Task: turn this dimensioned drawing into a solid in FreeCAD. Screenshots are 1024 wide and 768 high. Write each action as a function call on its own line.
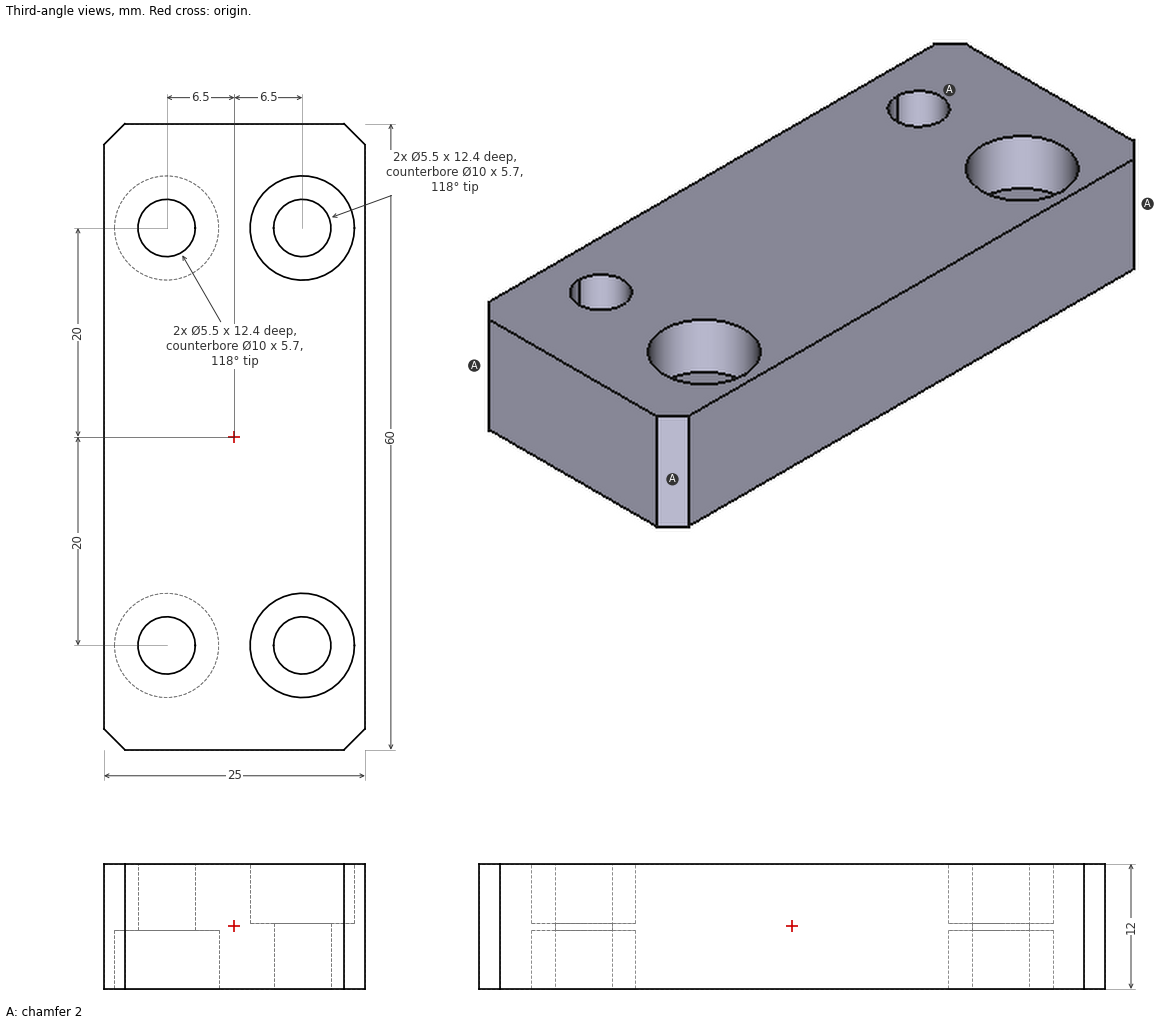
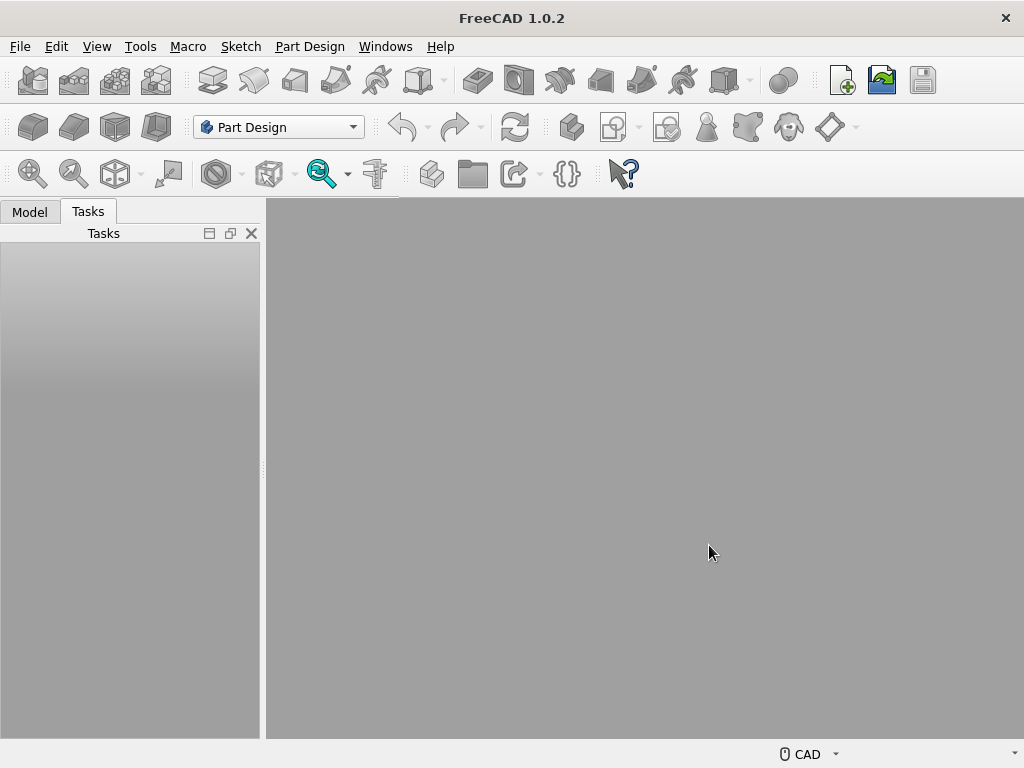
click(841, 80)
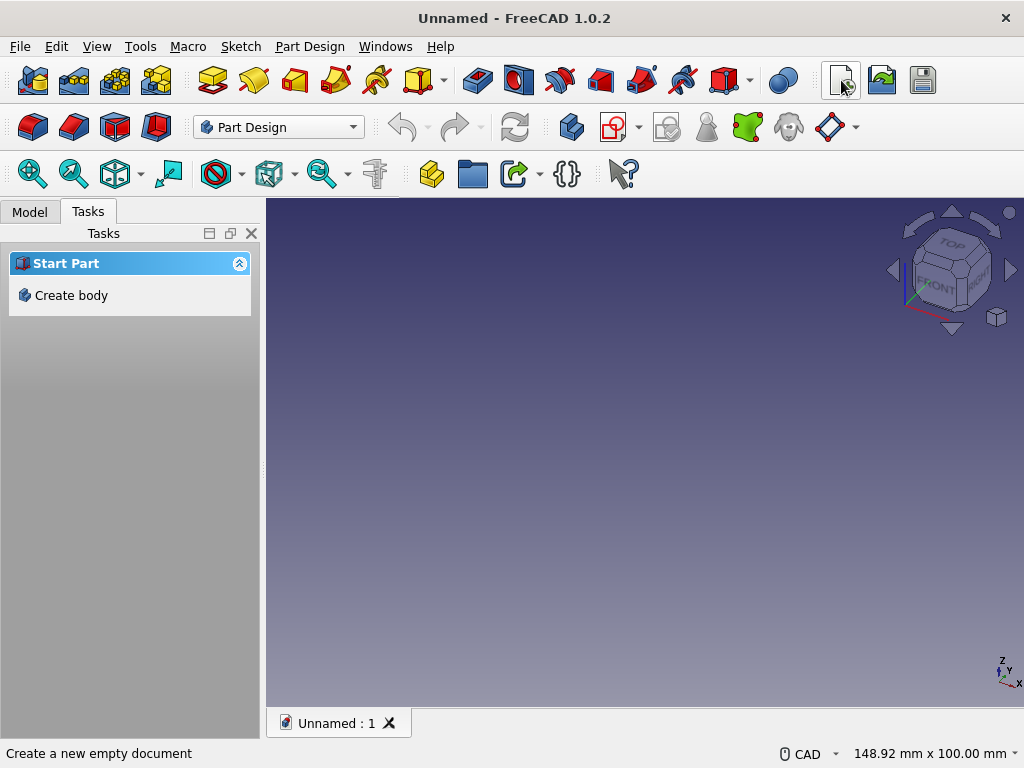
click(612, 128)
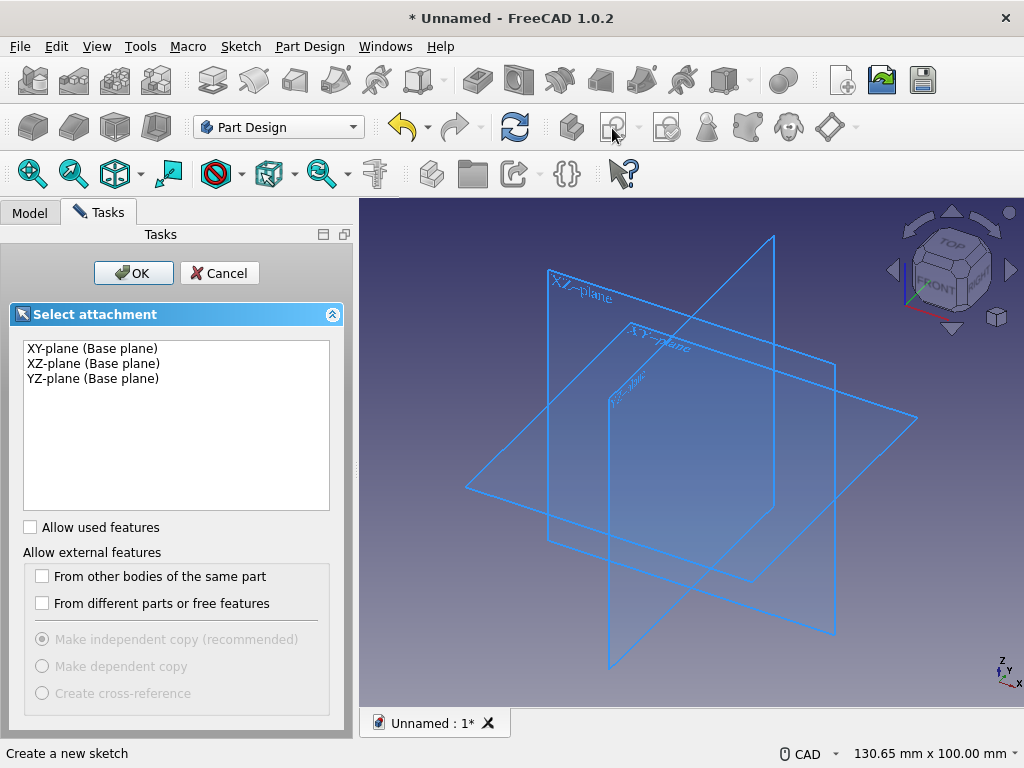
click(84, 348)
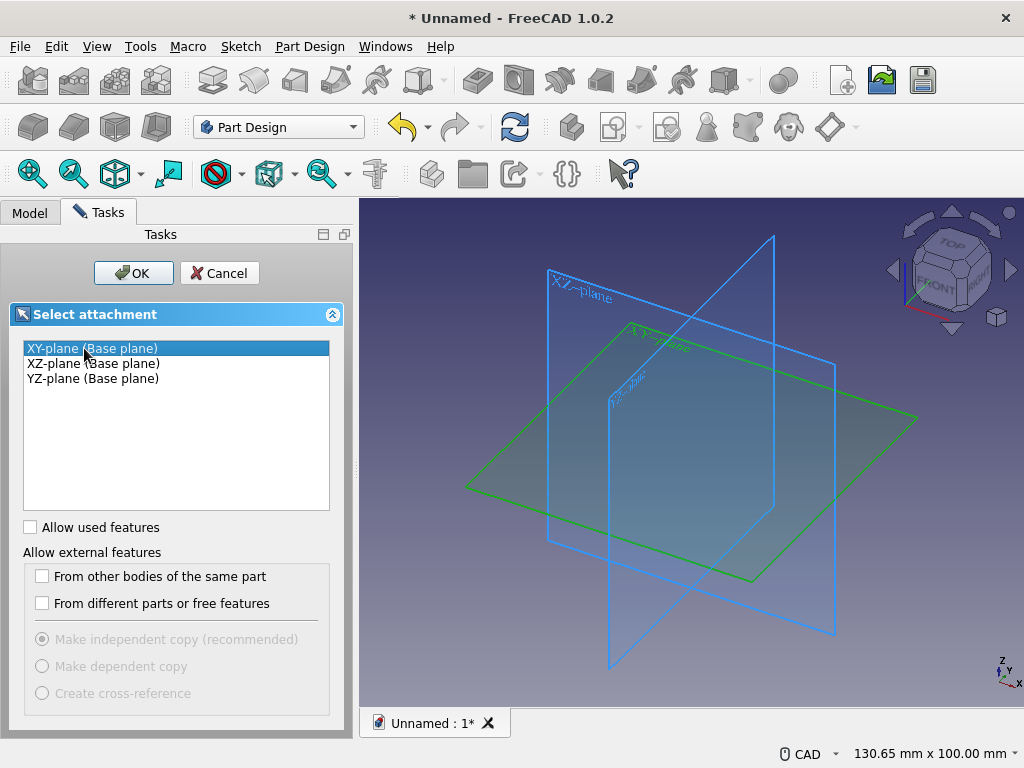
click(134, 273)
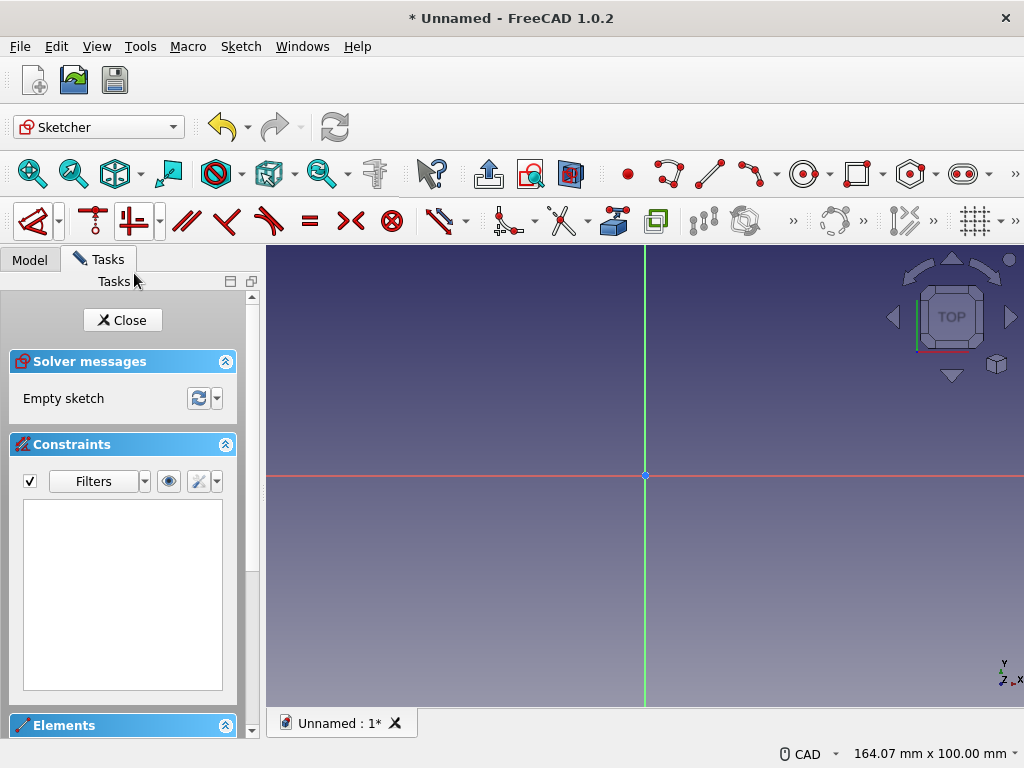
click(882, 174)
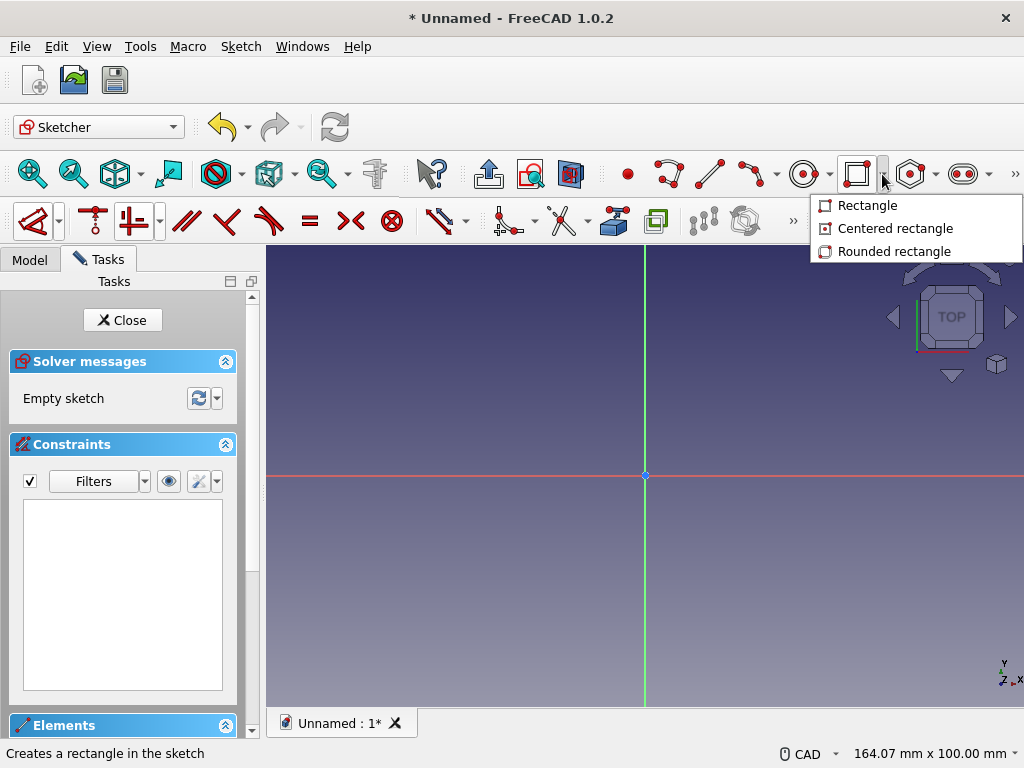
click(916, 228)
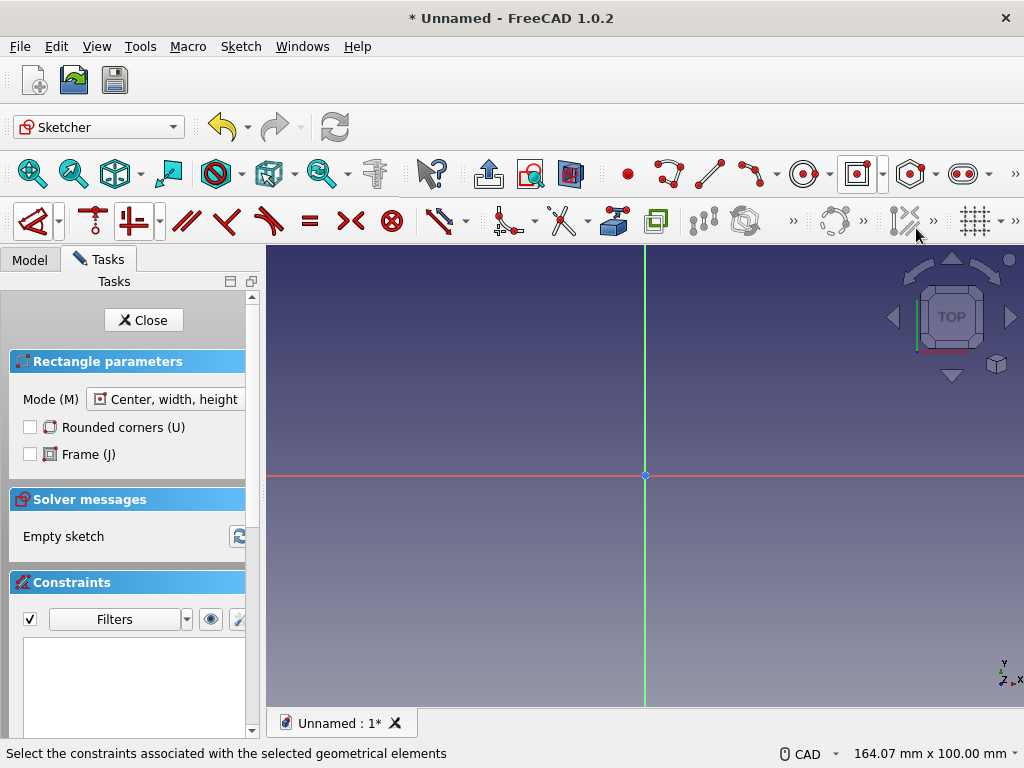
click(645, 476)
click(703, 337)
key(Escape)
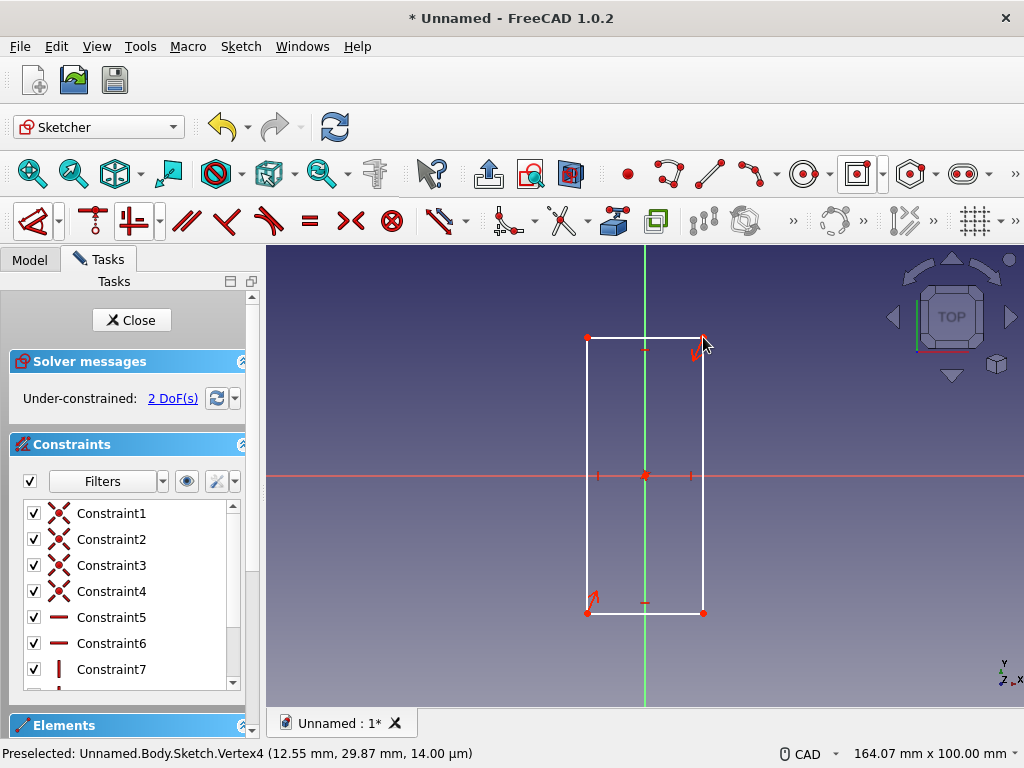
click(32, 222)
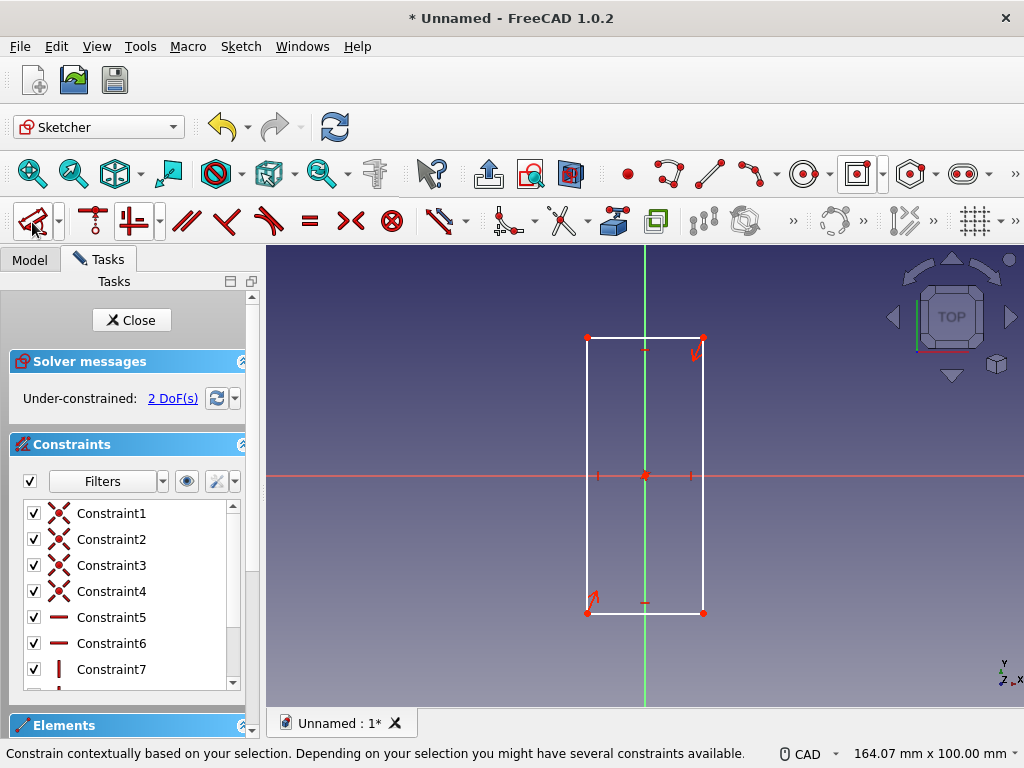
click(622, 614)
click(618, 648)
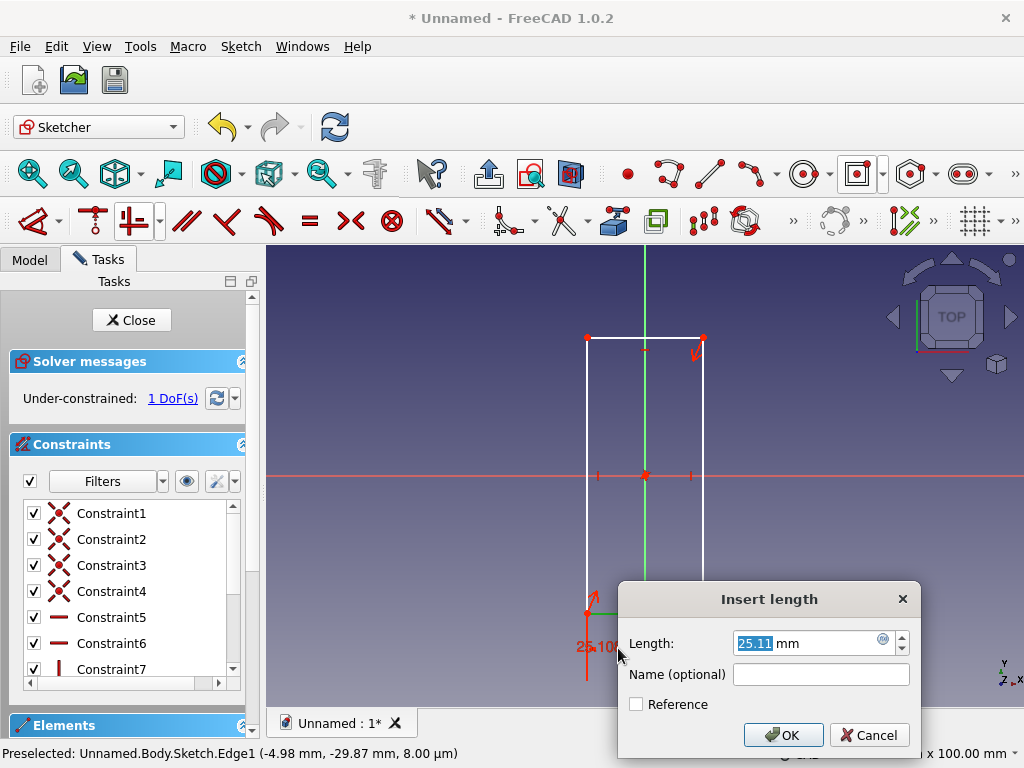
text(25)
key(Return)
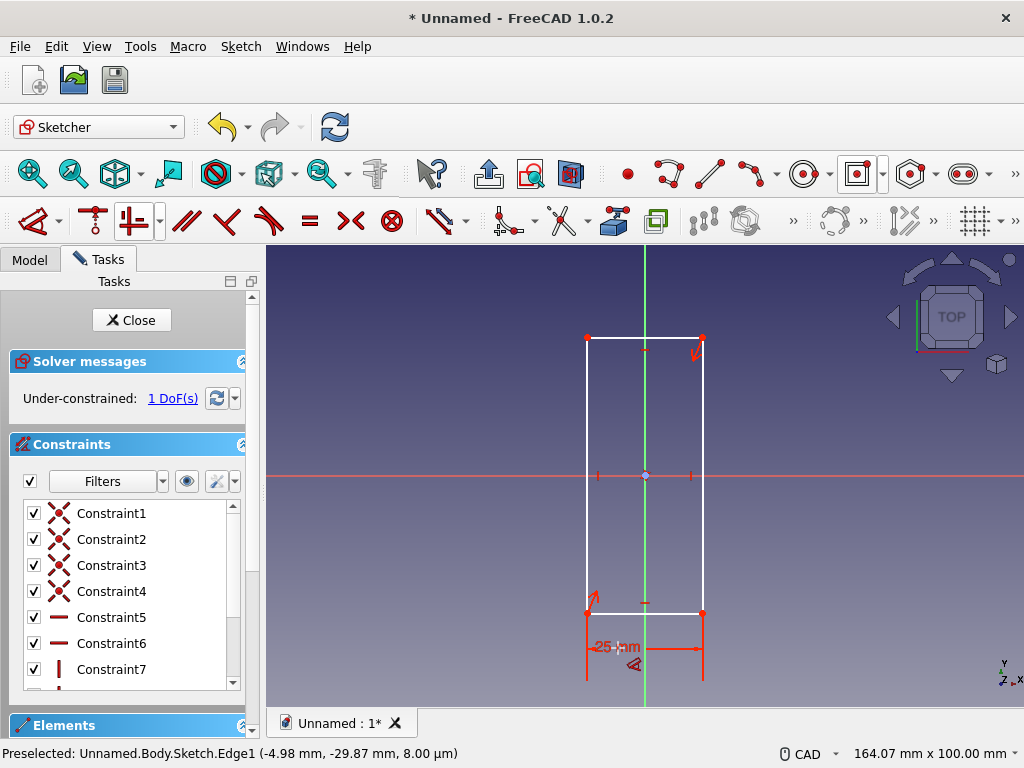
click(703, 531)
click(737, 413)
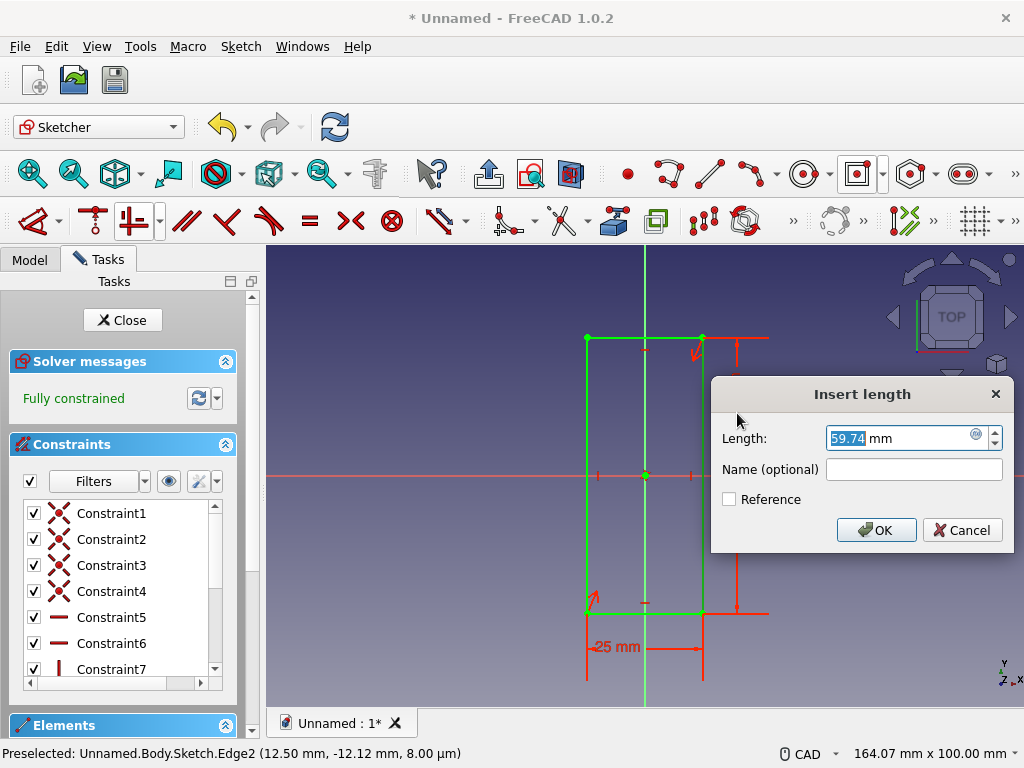
text(60)
key(Return)
key(Escape)